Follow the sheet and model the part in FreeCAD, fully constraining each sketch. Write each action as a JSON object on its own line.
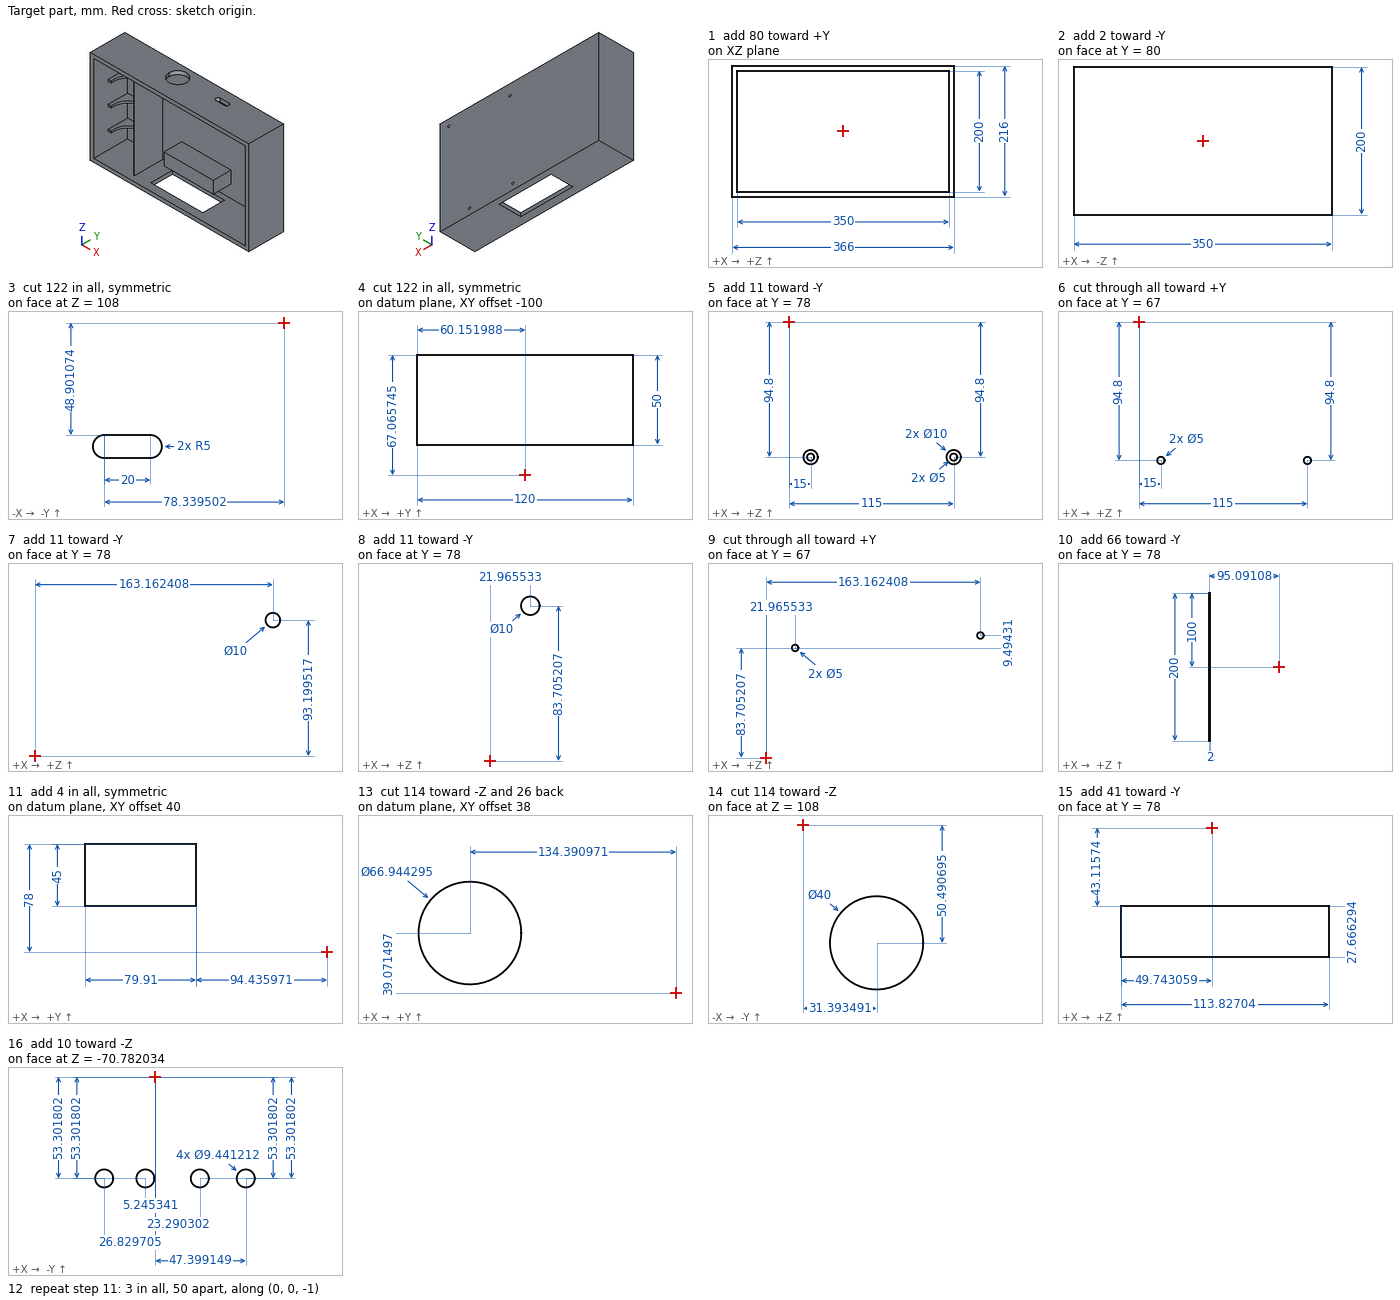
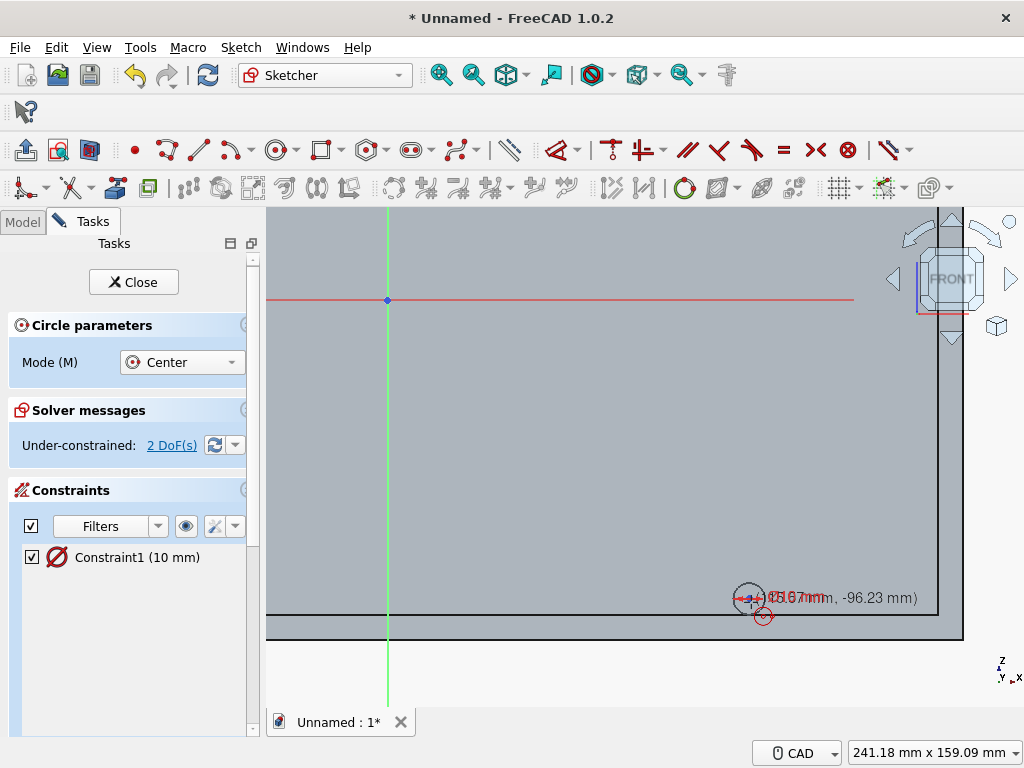
{"action": "scroll", "coordinate": [435, 598], "scroll_direction": "up", "scroll_amount": 2}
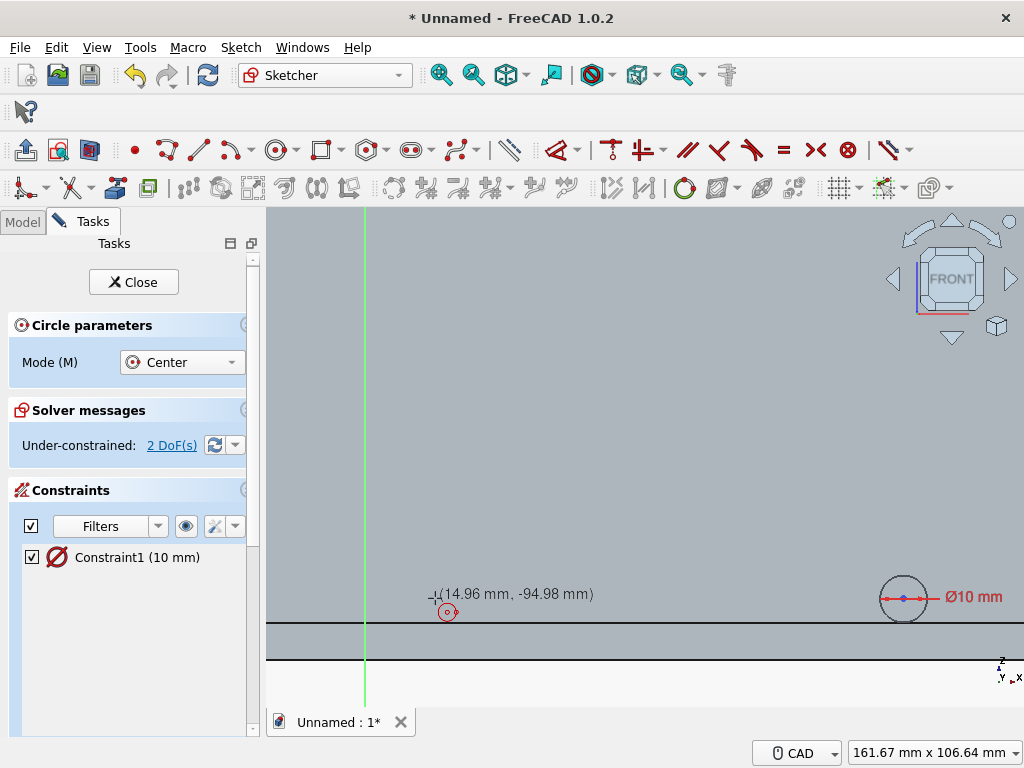
{"action": "left_click", "coordinate": [435, 598]}
{"action": "mouse_move", "coordinate": [452, 582]}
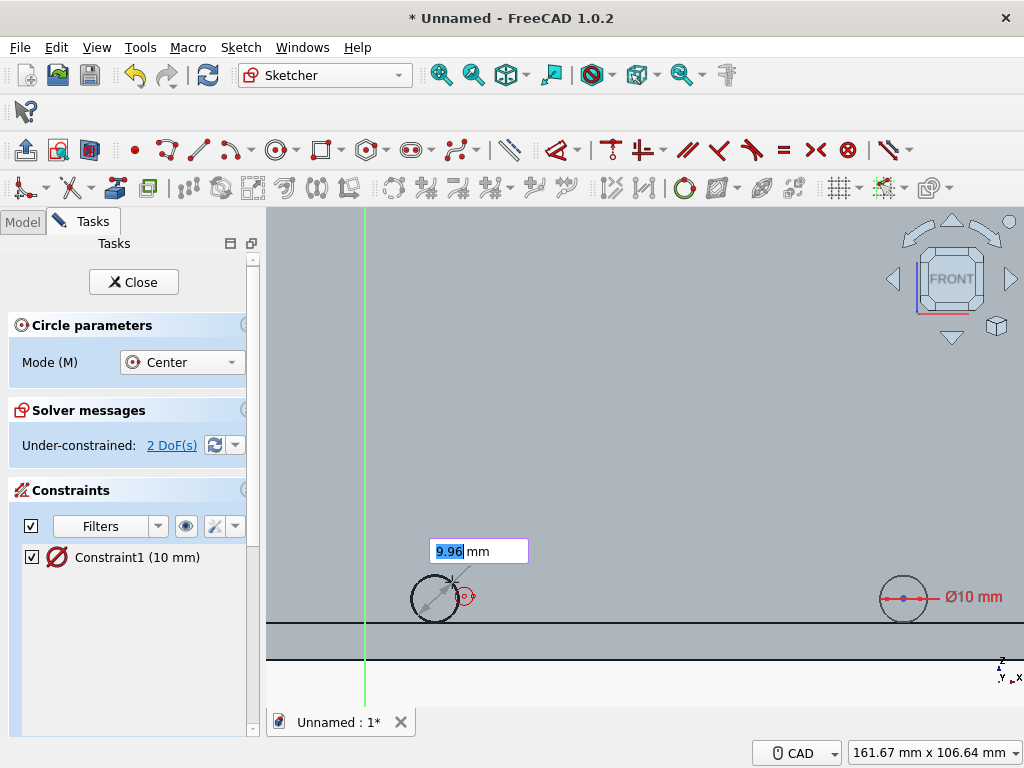
{"action": "type", "text": "10"}
{"action": "key", "text": "Return"}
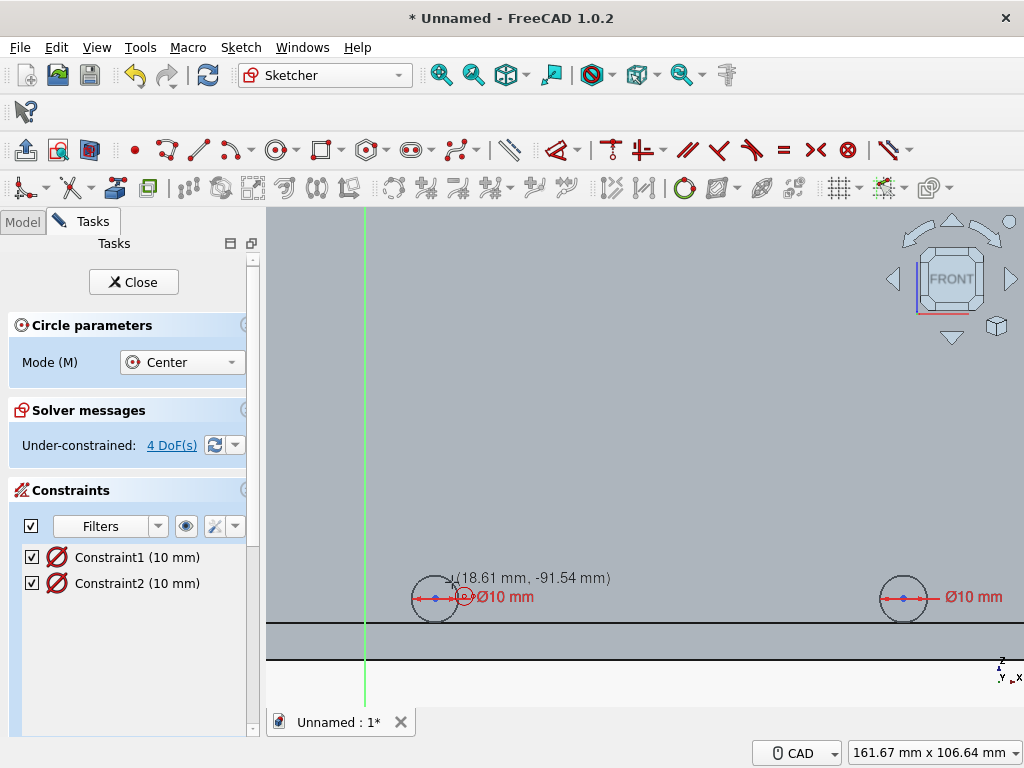
{"action": "scroll", "coordinate": [435, 598], "scroll_direction": "down", "scroll_amount": 2}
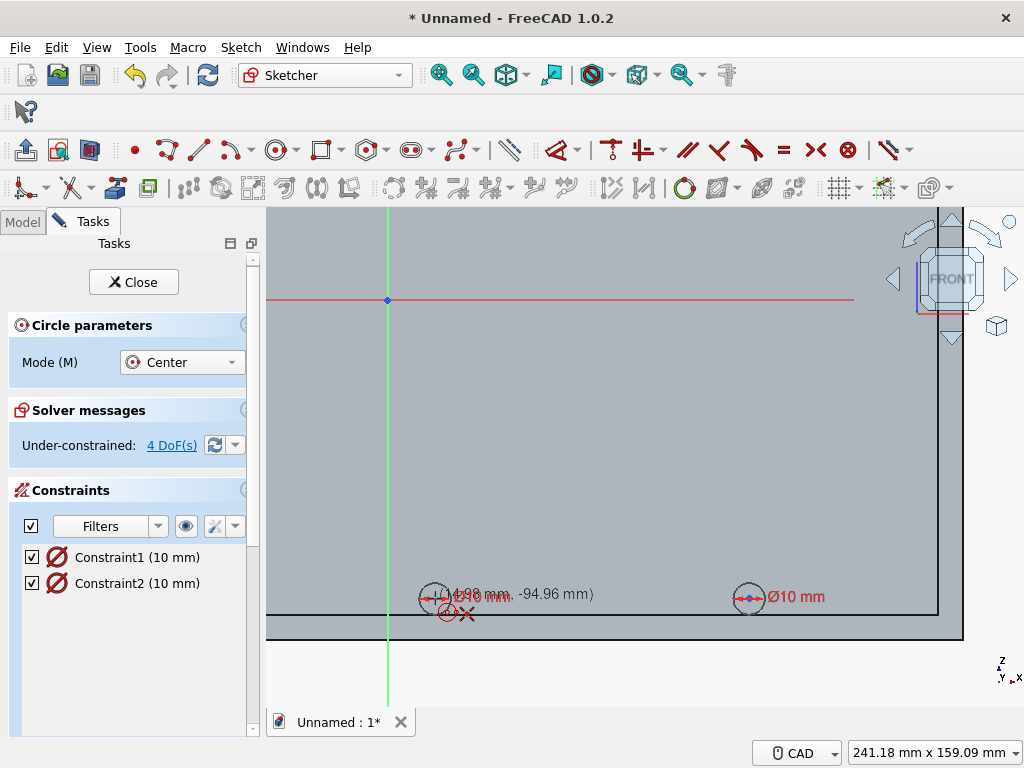
{"action": "scroll", "coordinate": [749, 598], "scroll_direction": "up", "scroll_amount": 6}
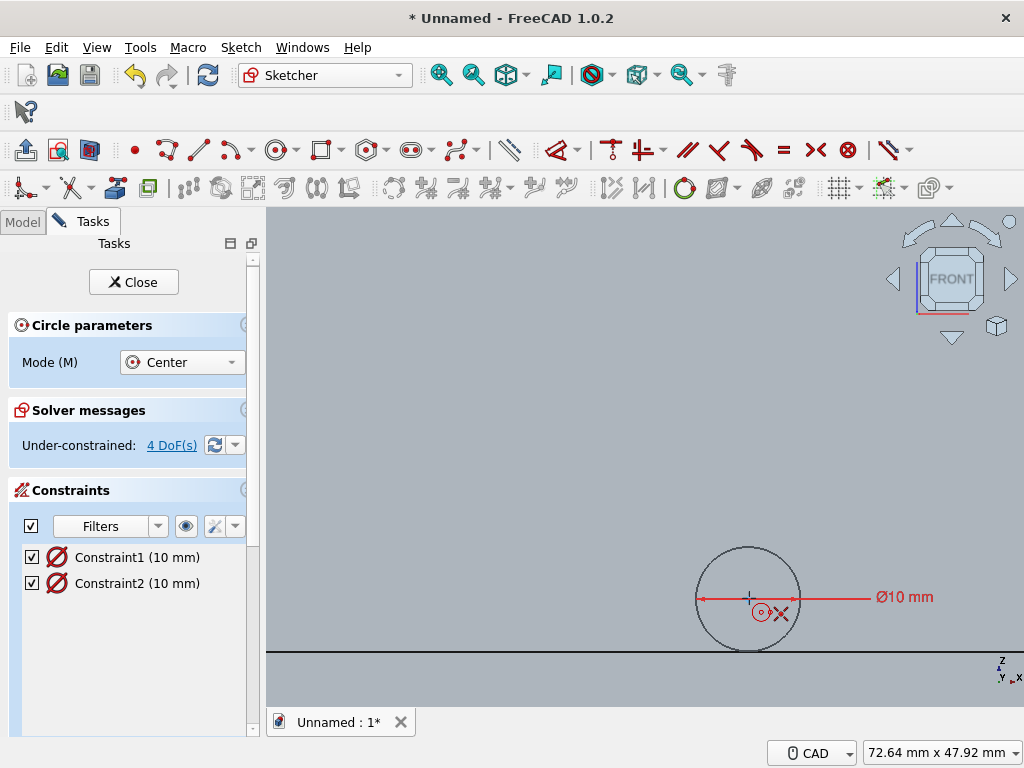
{"action": "left_click", "coordinate": [748, 599]}
{"action": "mouse_move", "coordinate": [767, 579]}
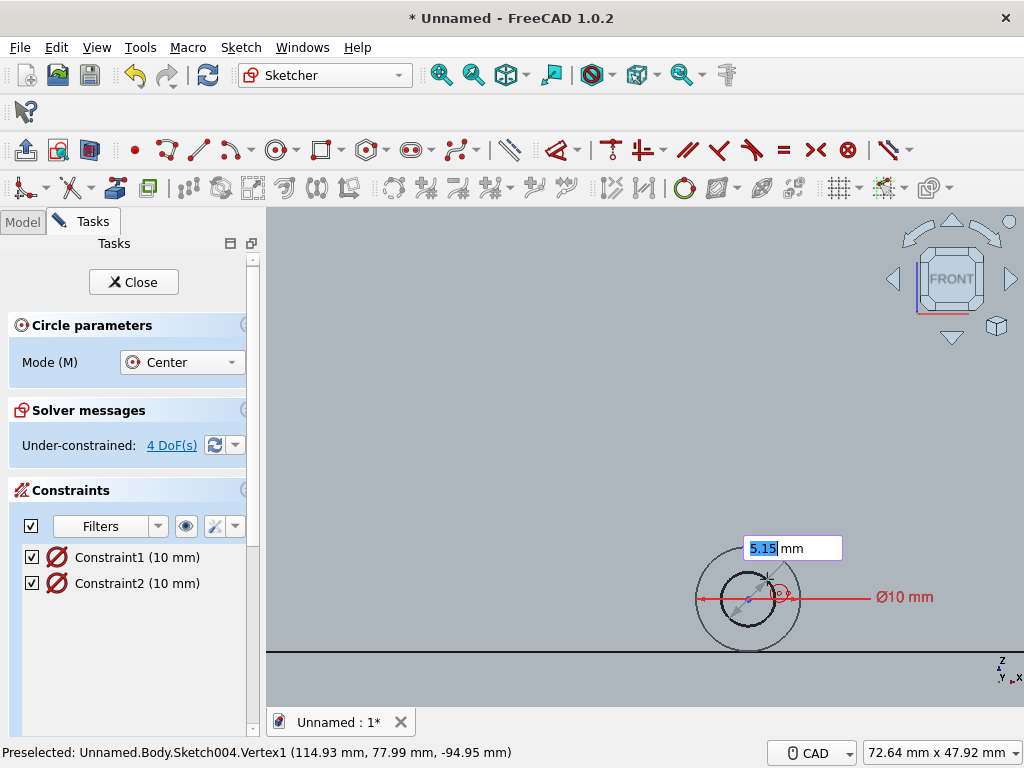
{"action": "type", "text": "5"}
{"action": "key", "text": "Return"}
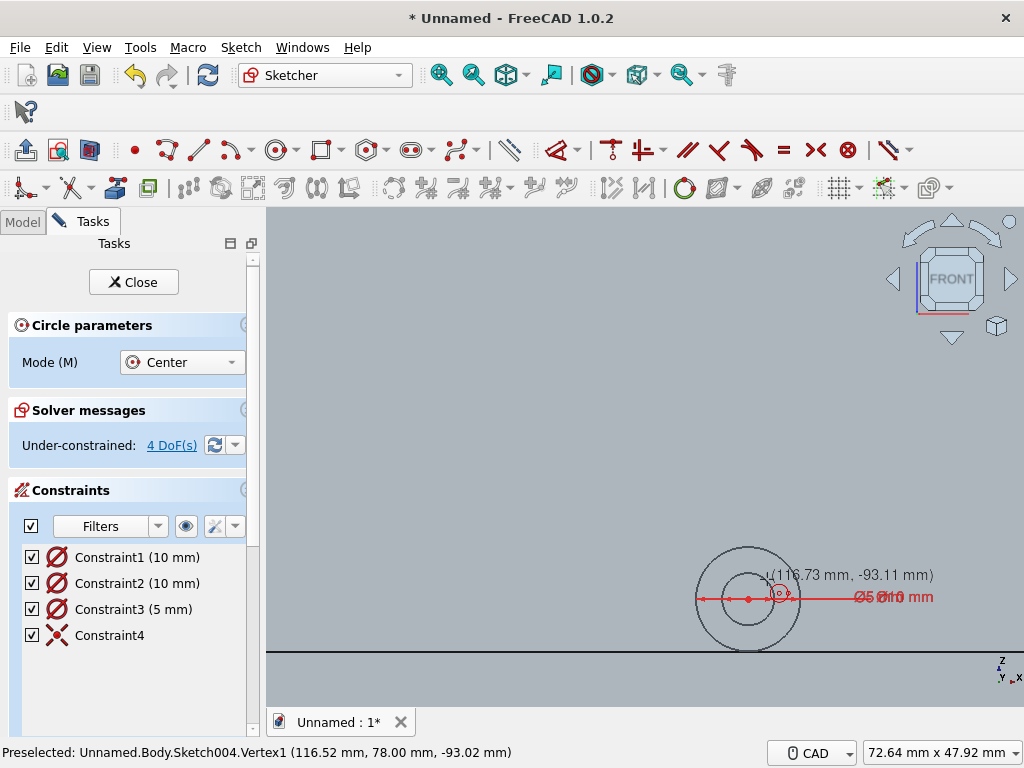
{"action": "scroll", "coordinate": [750, 598], "scroll_direction": "down", "scroll_amount": 6}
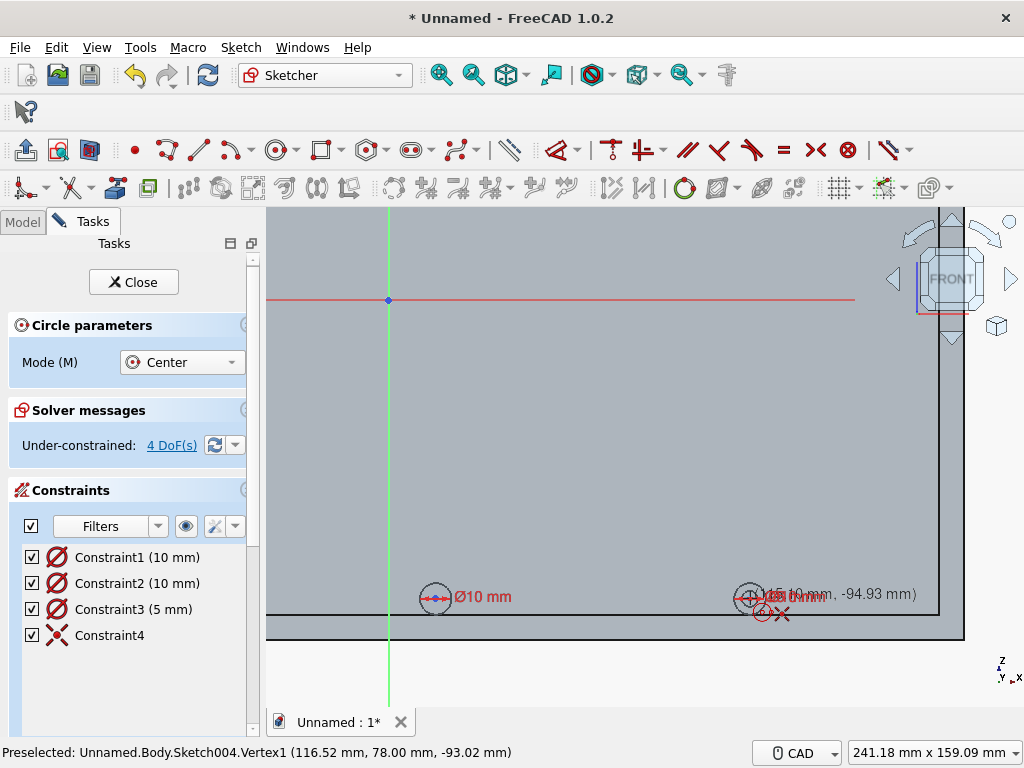
{"action": "scroll", "coordinate": [436, 598], "scroll_direction": "up", "scroll_amount": 6}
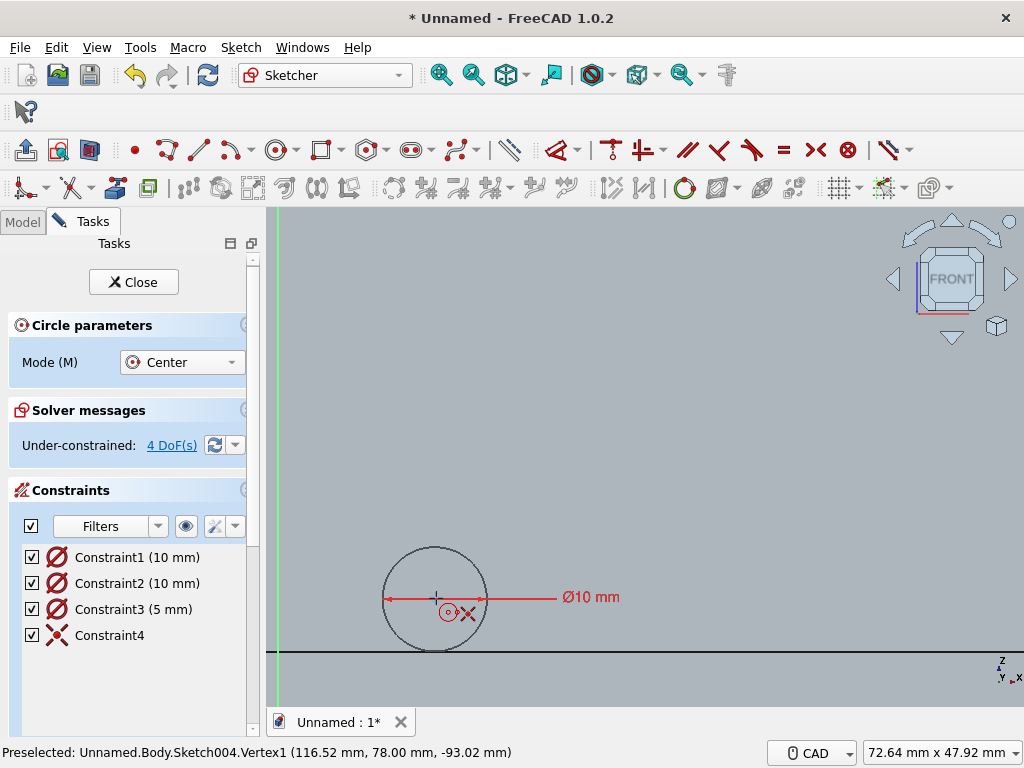
{"action": "left_click", "coordinate": [435, 599]}
{"action": "mouse_move", "coordinate": [453, 579]}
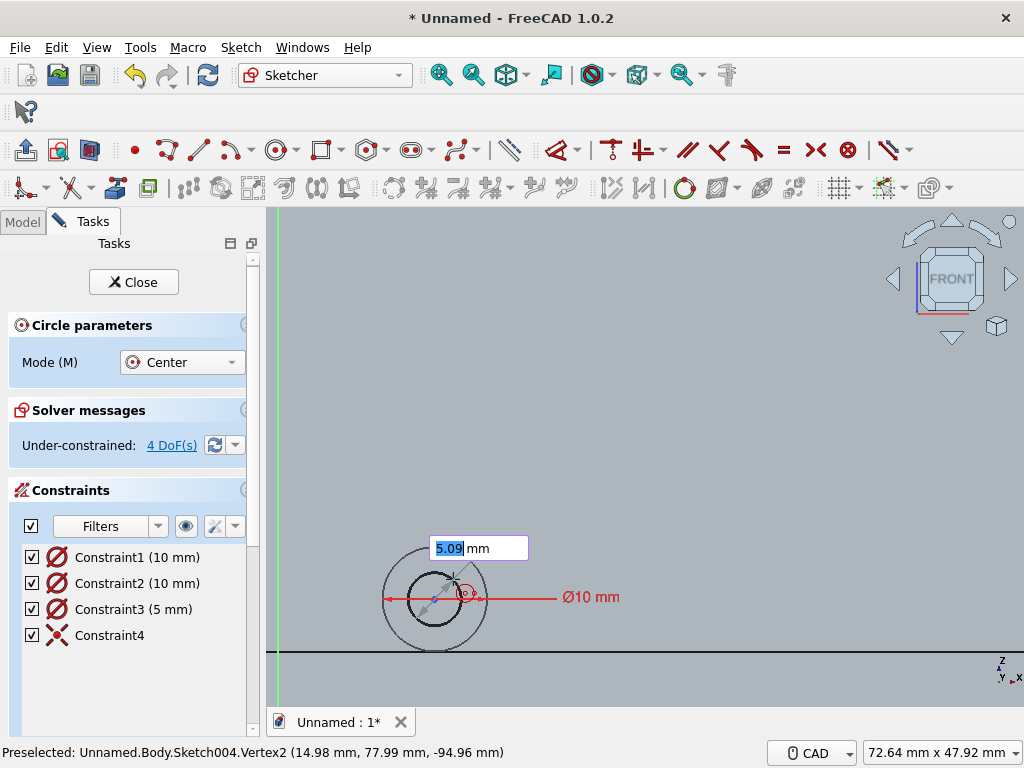
{"action": "type", "text": "5"}
{"action": "key", "text": "Return"}
{"action": "key", "text": "Escape"}